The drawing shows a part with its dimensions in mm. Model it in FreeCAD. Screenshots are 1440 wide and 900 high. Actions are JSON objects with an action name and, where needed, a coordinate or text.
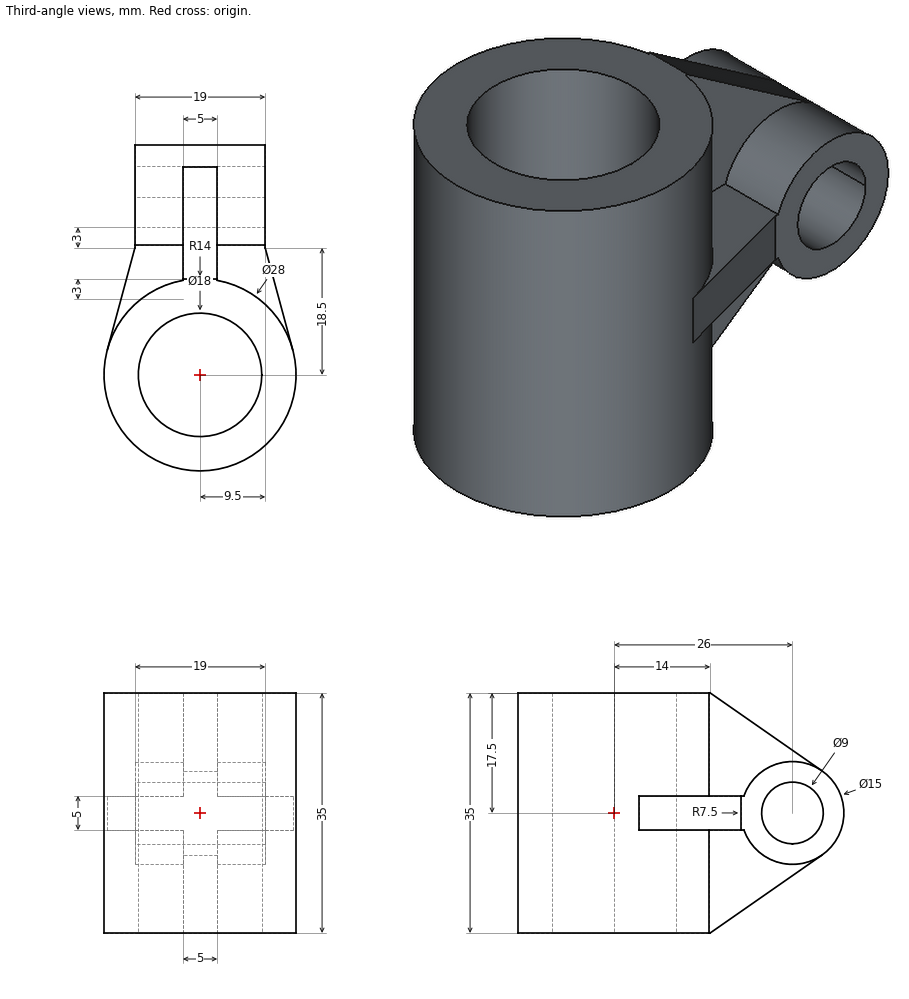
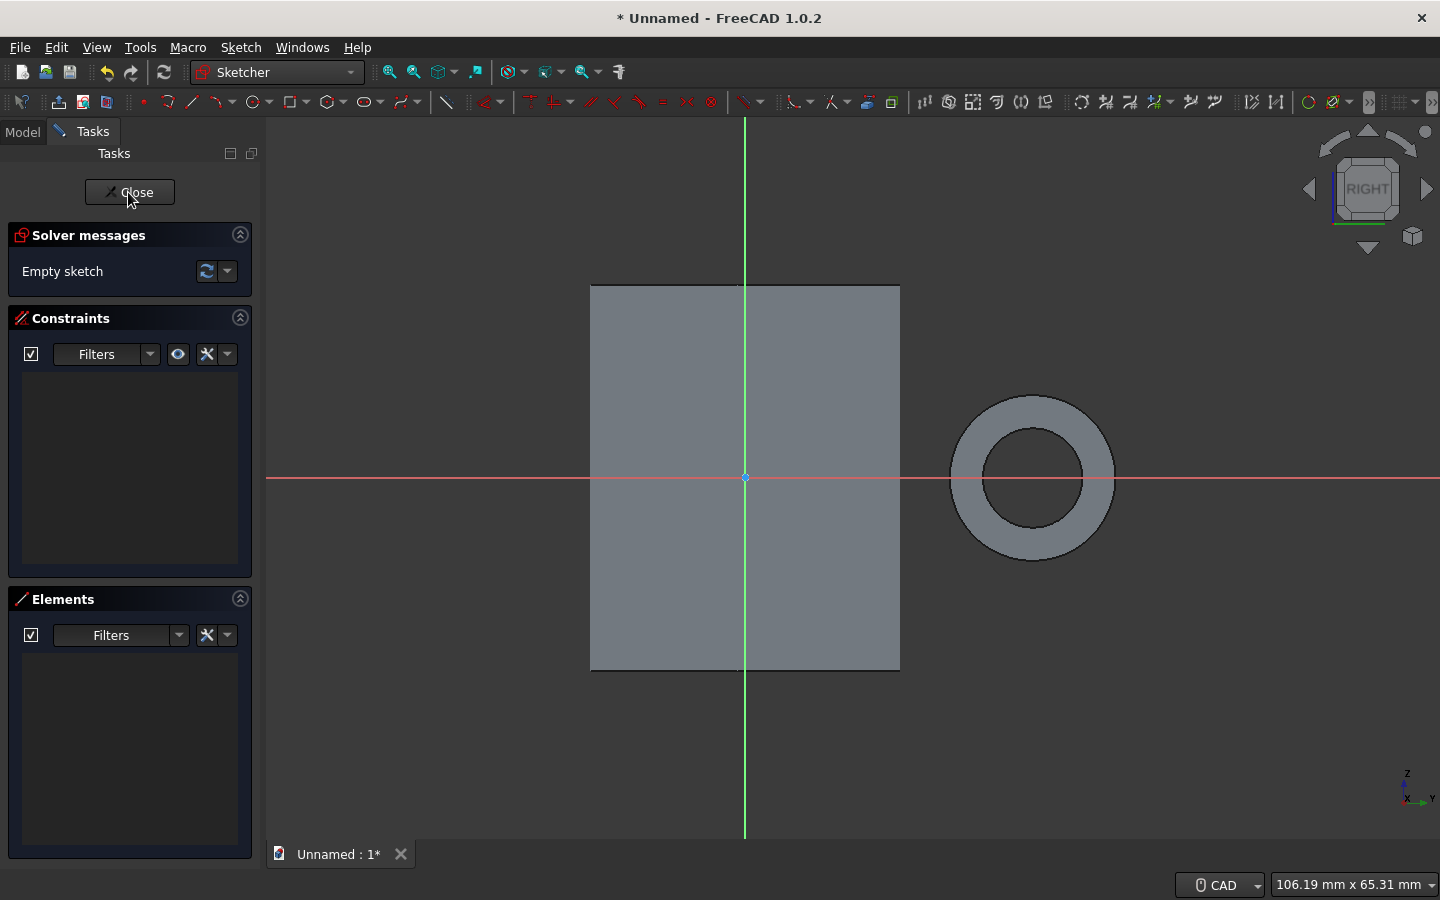
{"action": "key", "text": "g m"}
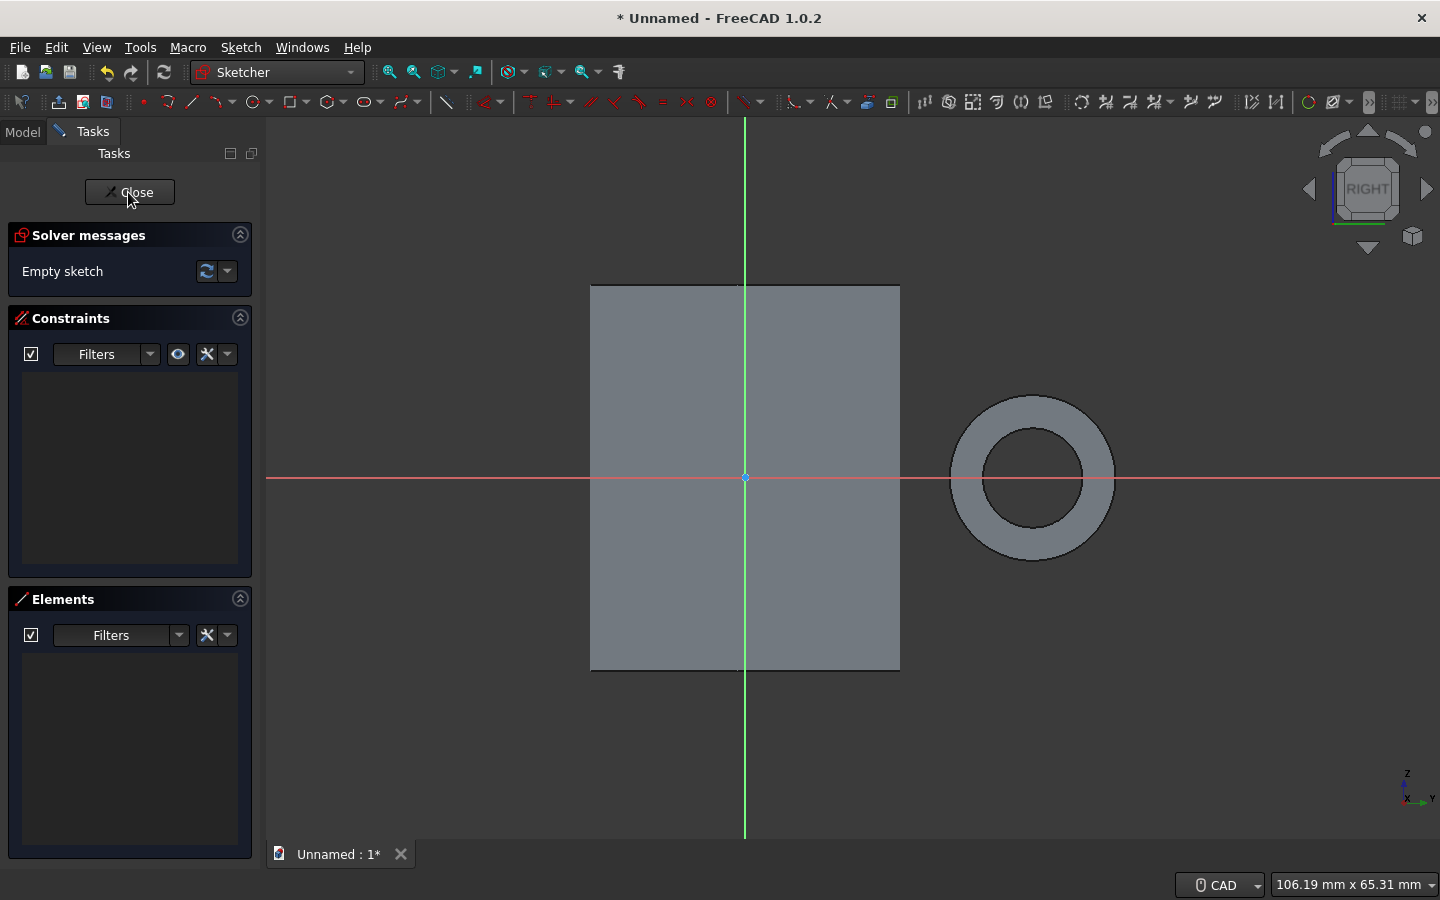
{"action": "left_click", "coordinate": [1080, 410]}
{"action": "left_click", "coordinate": [900, 285]}
{"action": "left_click", "coordinate": [900, 671]}
{"action": "left_click", "coordinate": [1080, 546]}
{"action": "right_click", "coordinate": [1080, 546]}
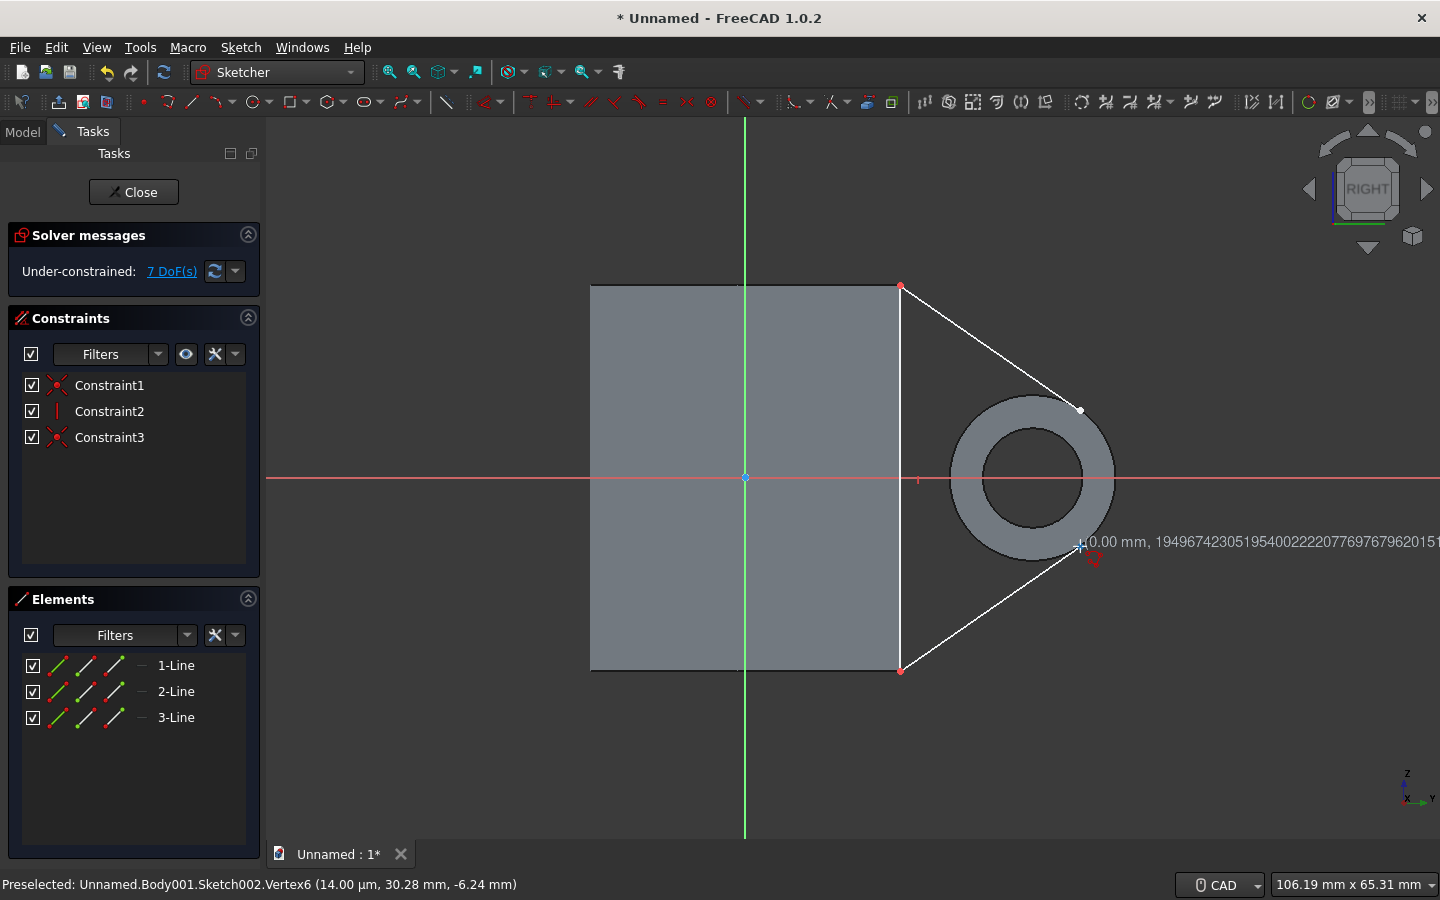
{"action": "left_click", "coordinate": [216, 102]}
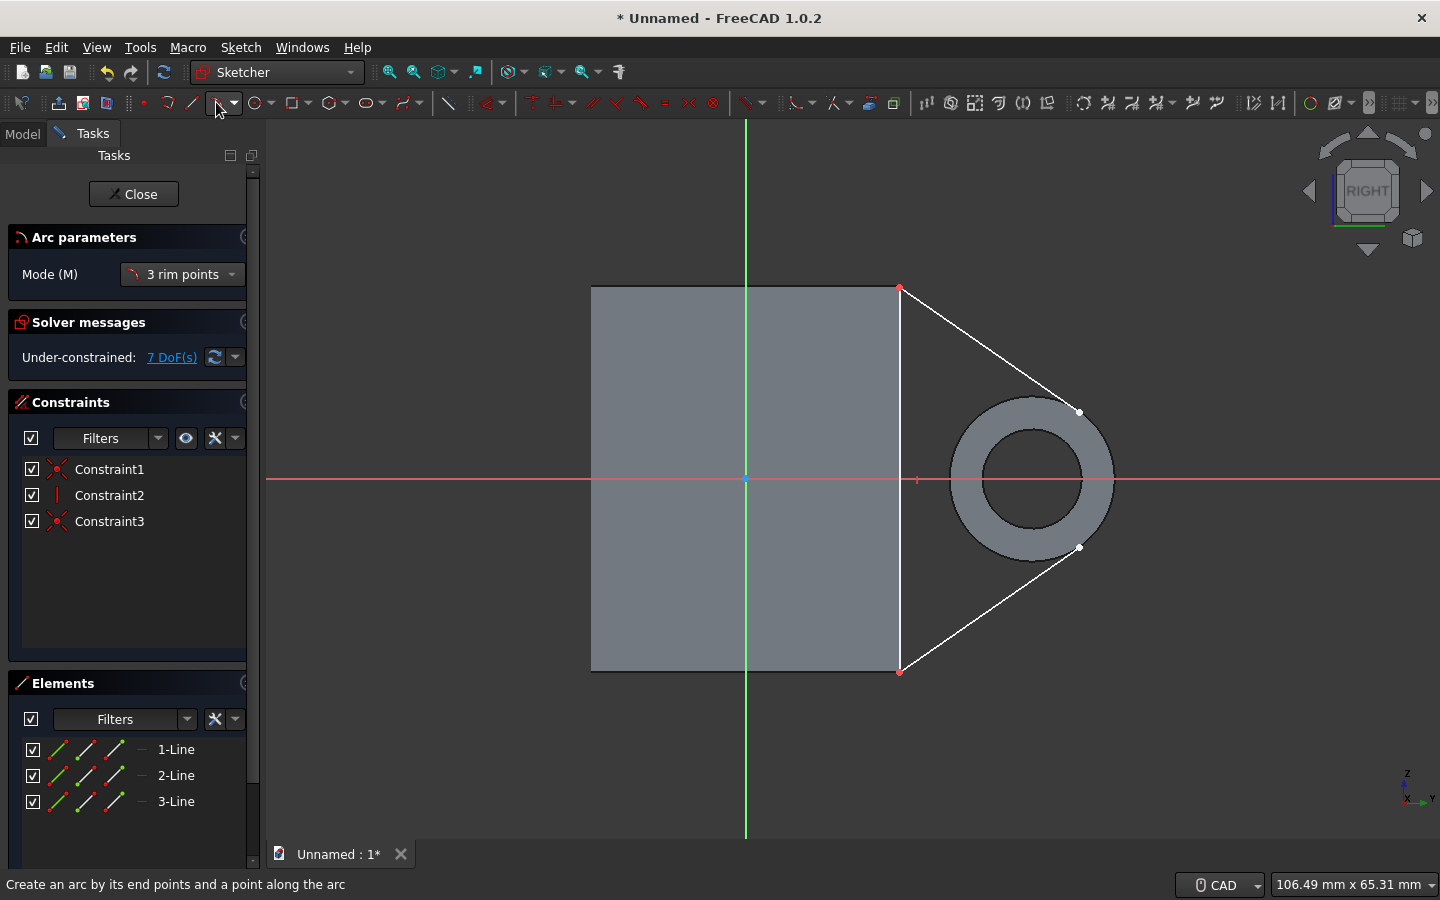
{"action": "left_click", "coordinate": [1079, 548]}
{"action": "left_click", "coordinate": [1079, 412]}
{"action": "left_click", "coordinate": [957, 444]}
{"action": "key", "text": "Escape"}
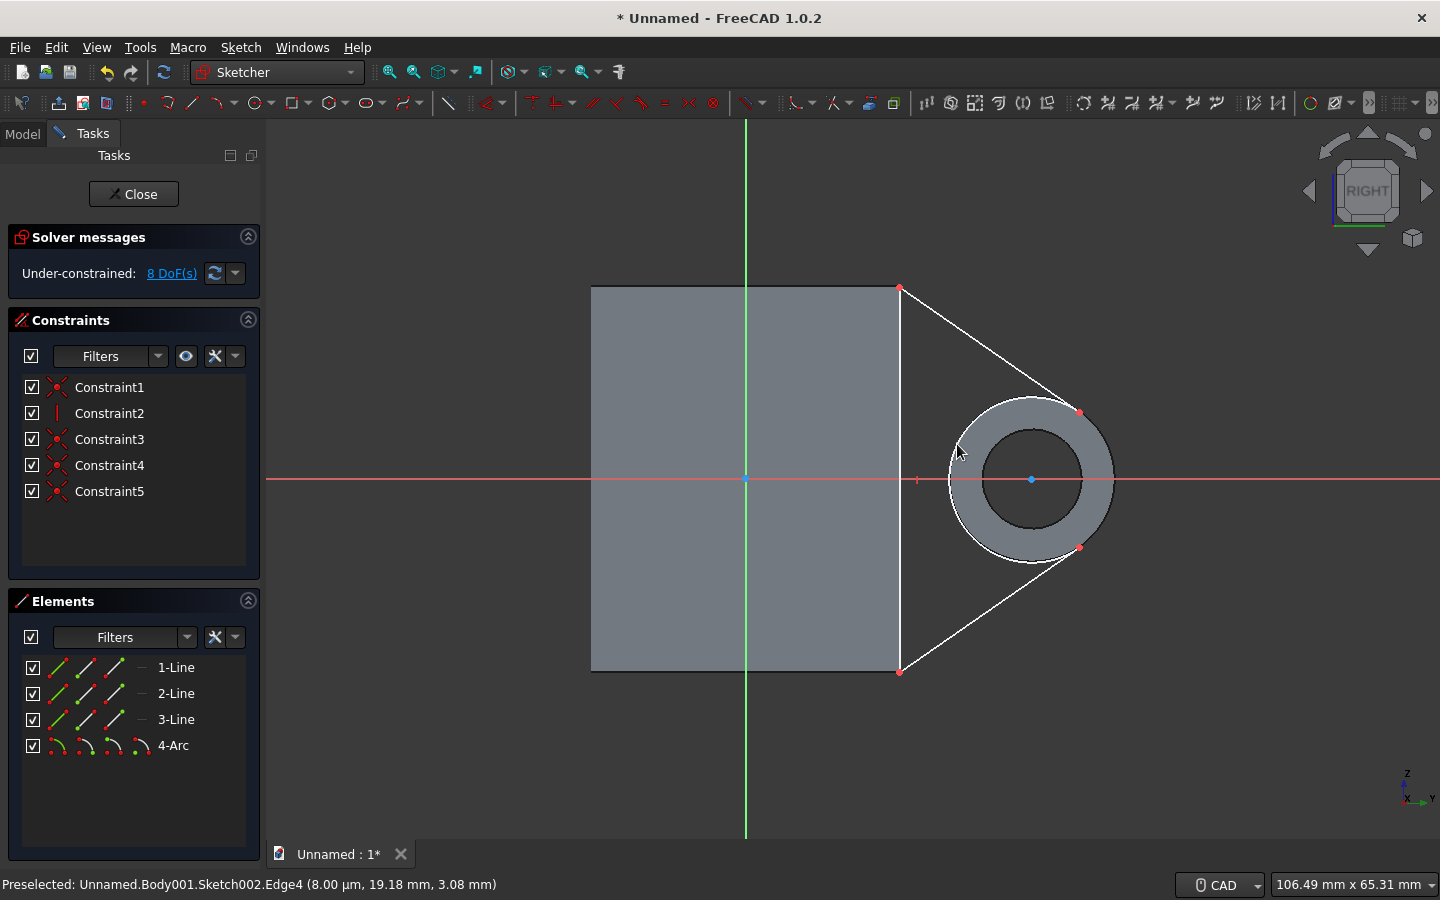
{"action": "left_click", "coordinate": [1026, 375]}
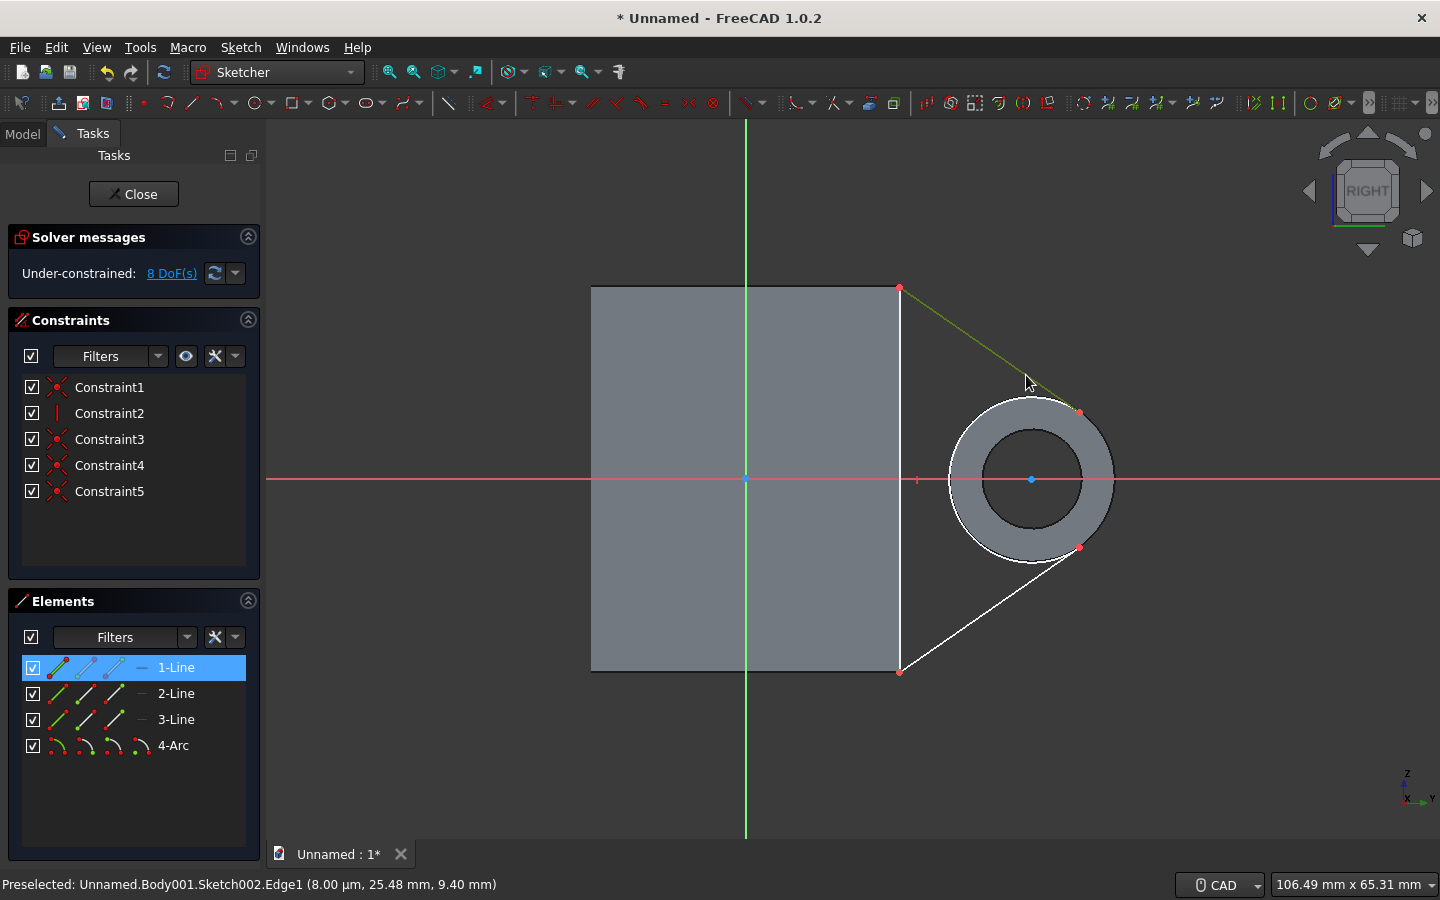
{"action": "left_click", "coordinate": [979, 417]}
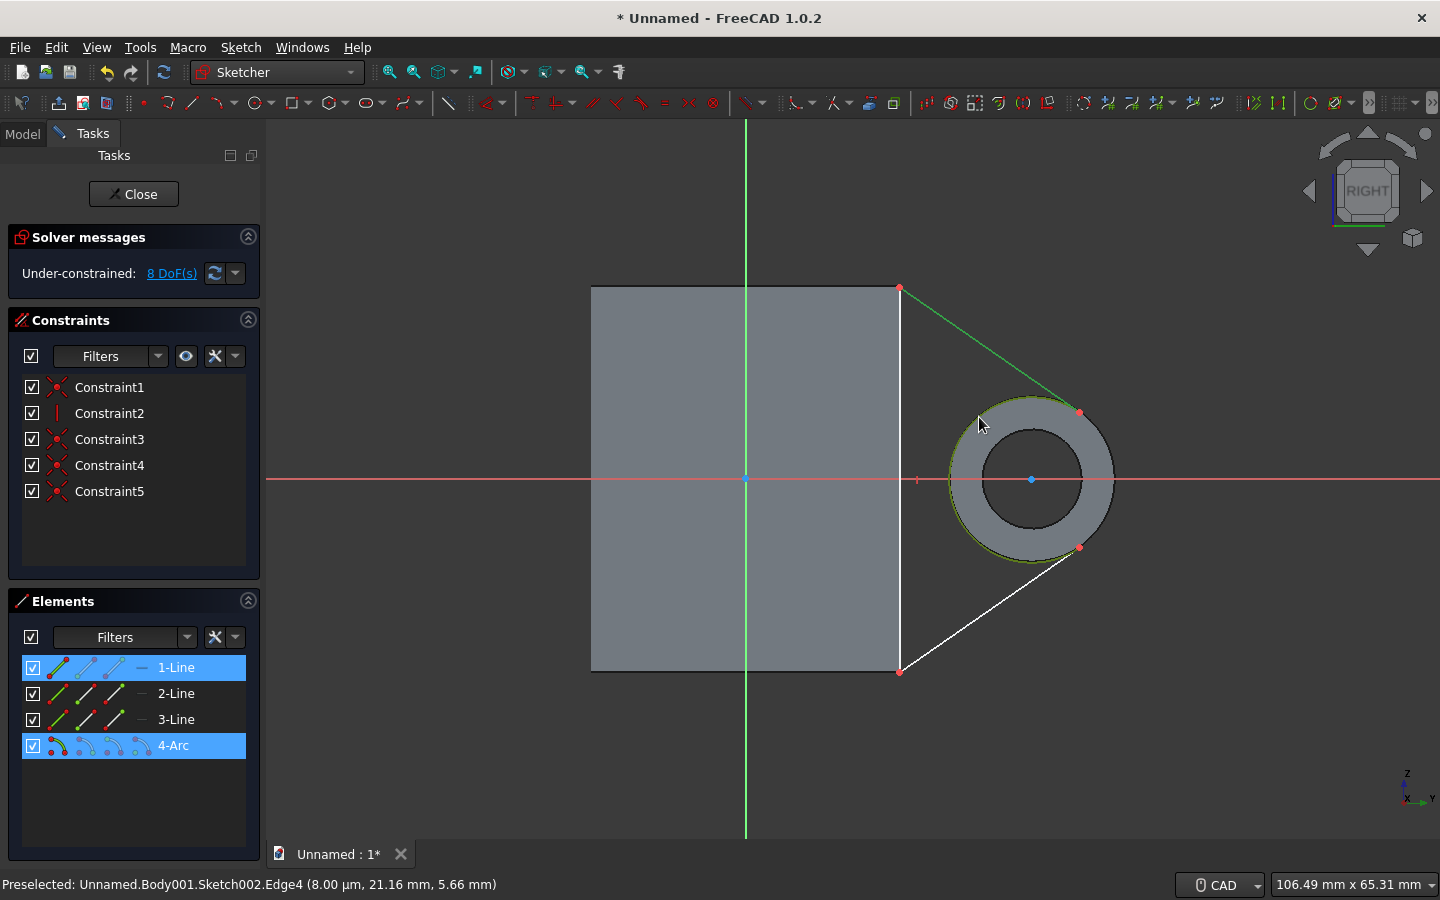
{"action": "key", "text": "t"}